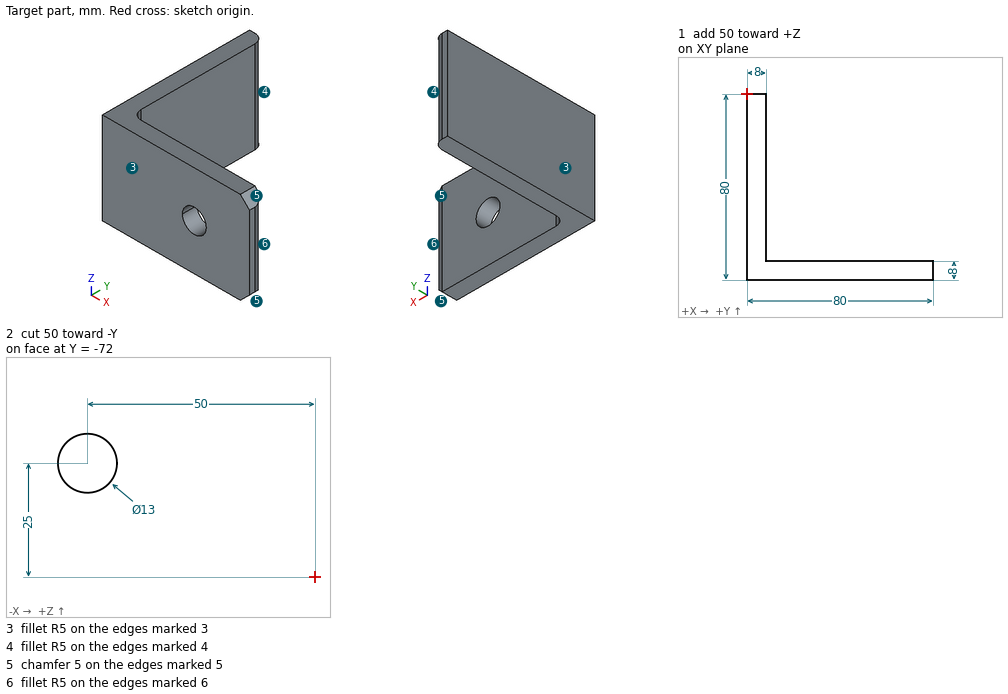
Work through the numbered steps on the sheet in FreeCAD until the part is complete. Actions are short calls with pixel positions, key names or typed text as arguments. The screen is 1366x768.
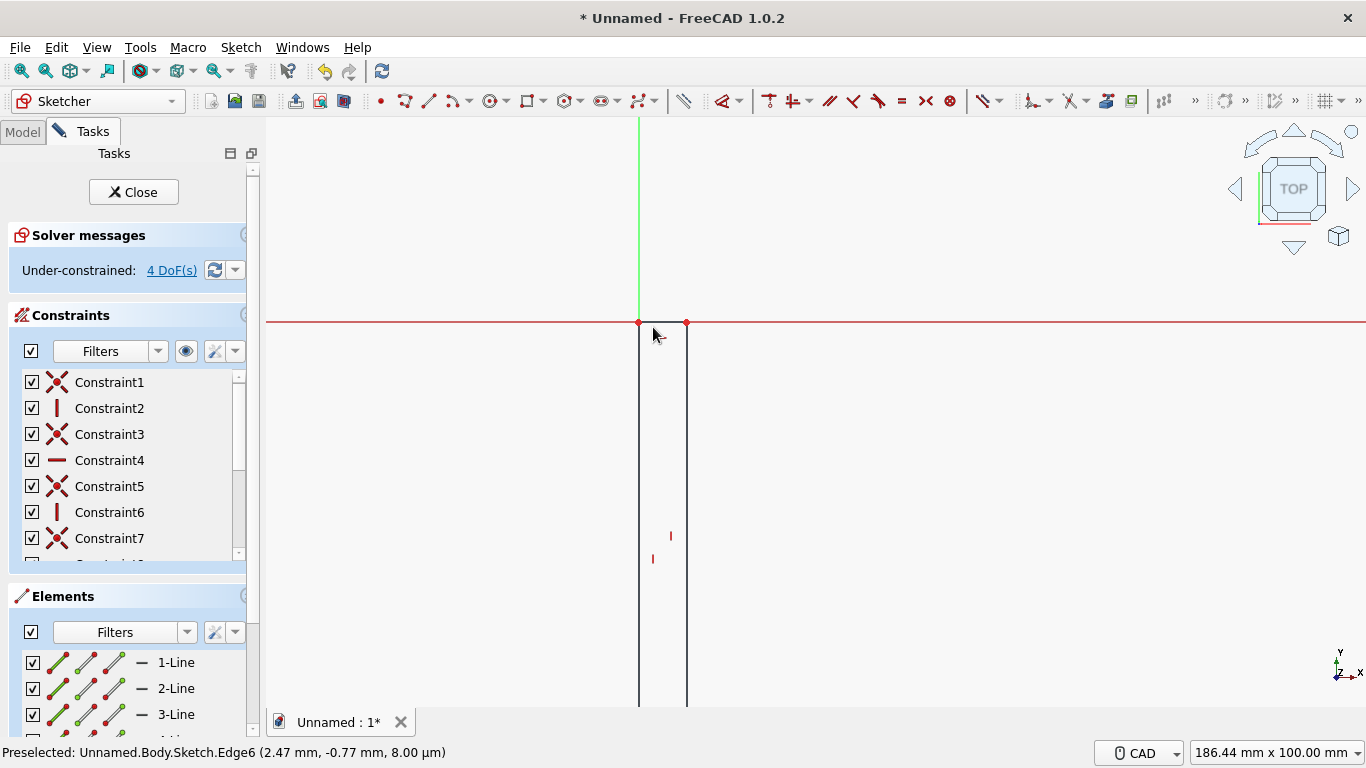
scroll(489, 145, down, 2)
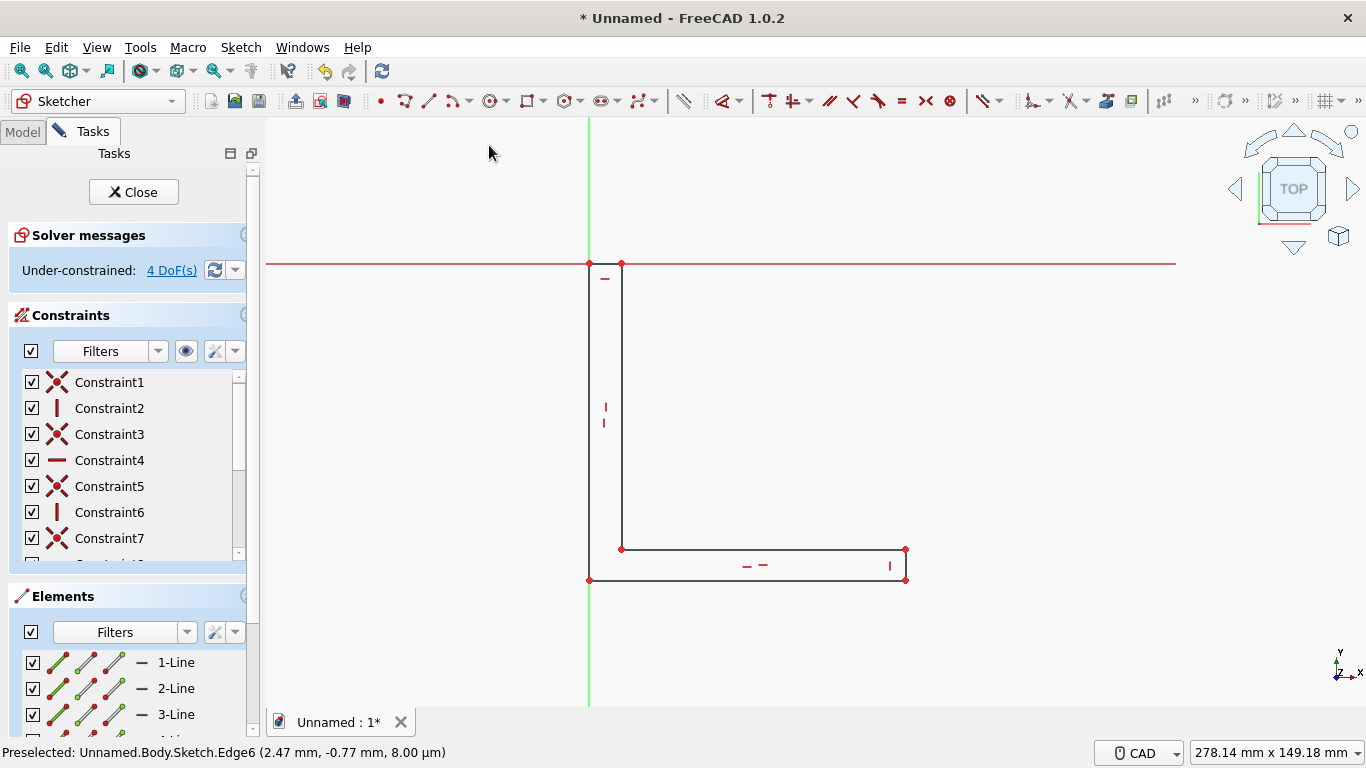
scroll(906, 572, up, 2)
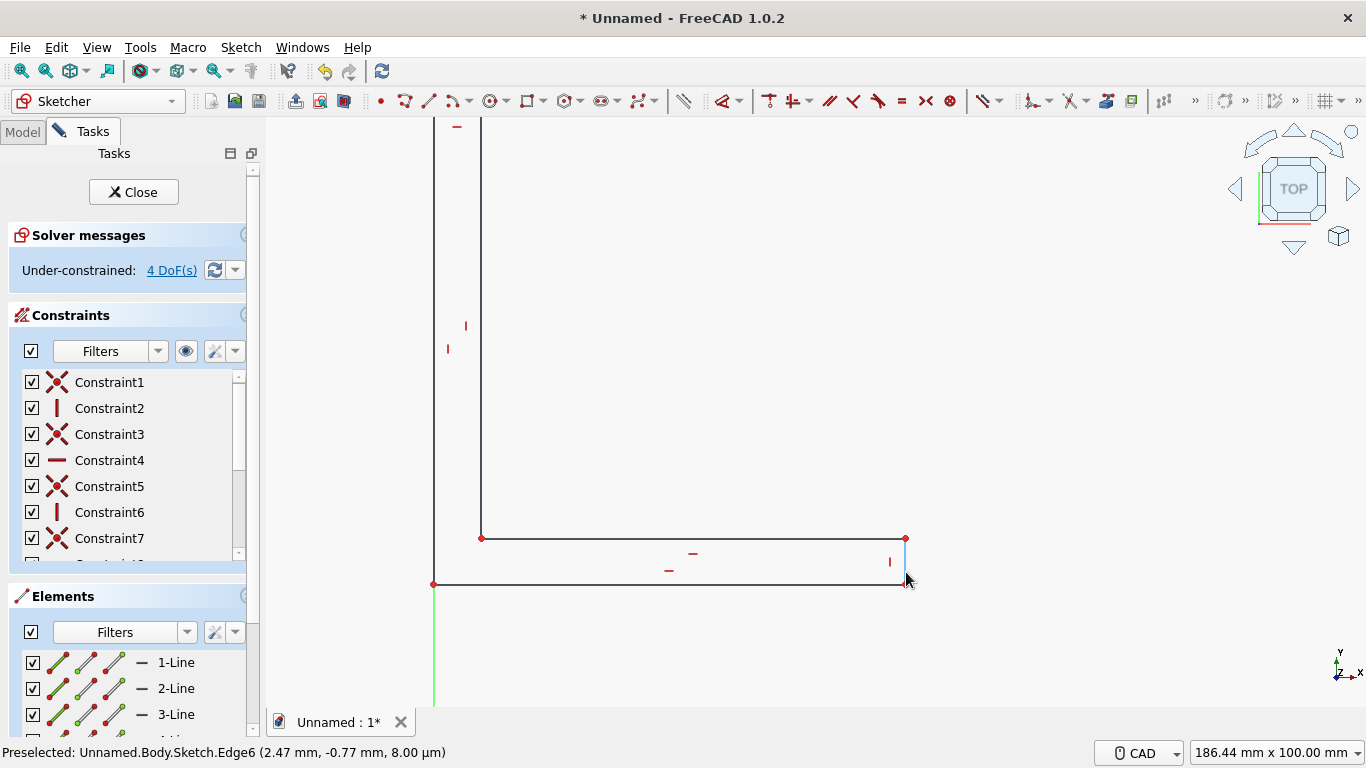
click(905, 571)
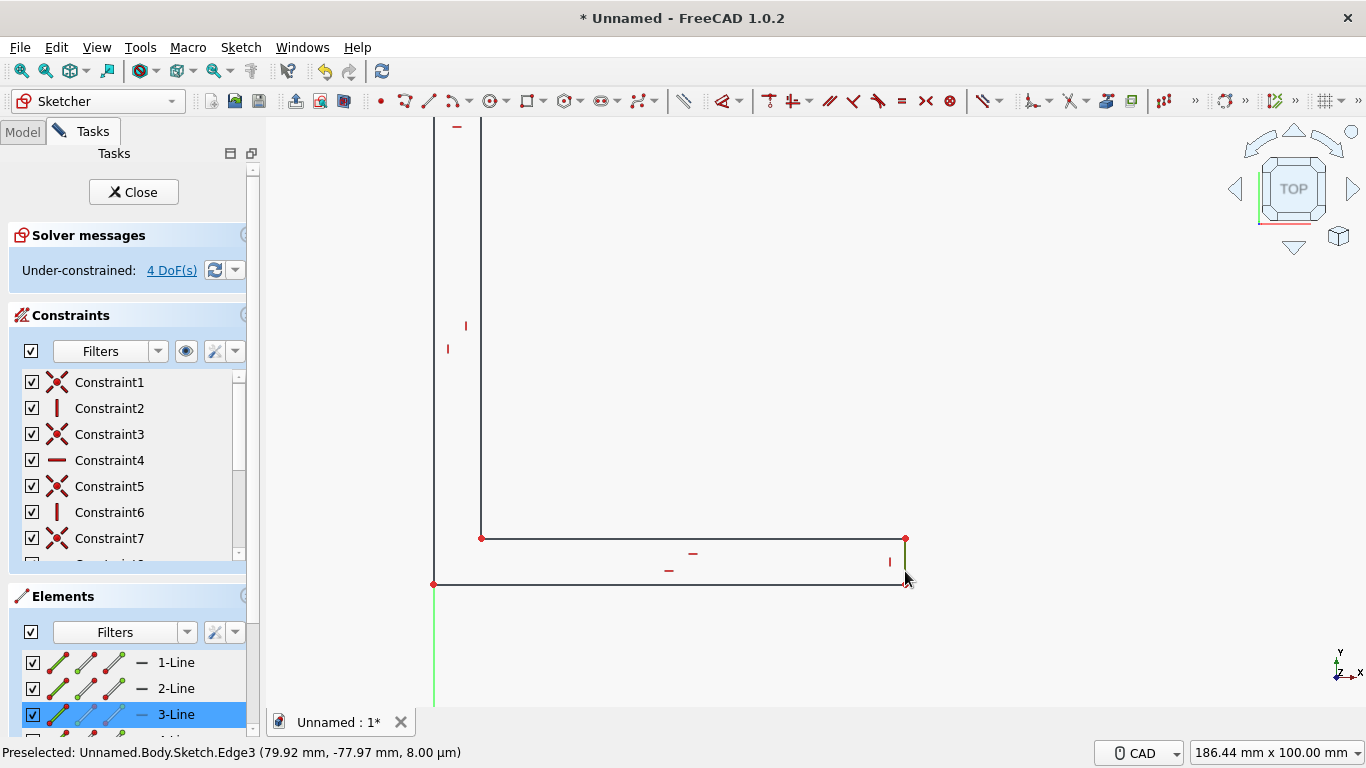
click(742, 102)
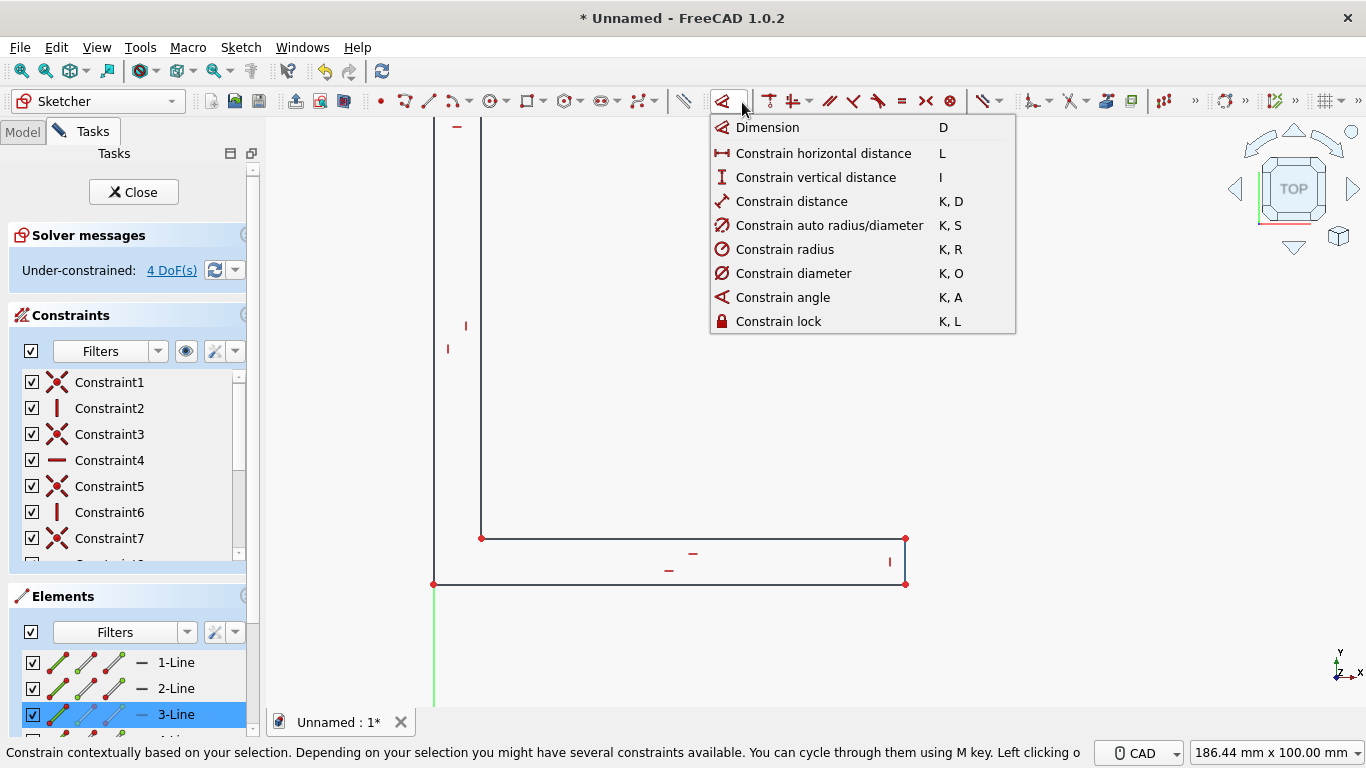
click(863, 177)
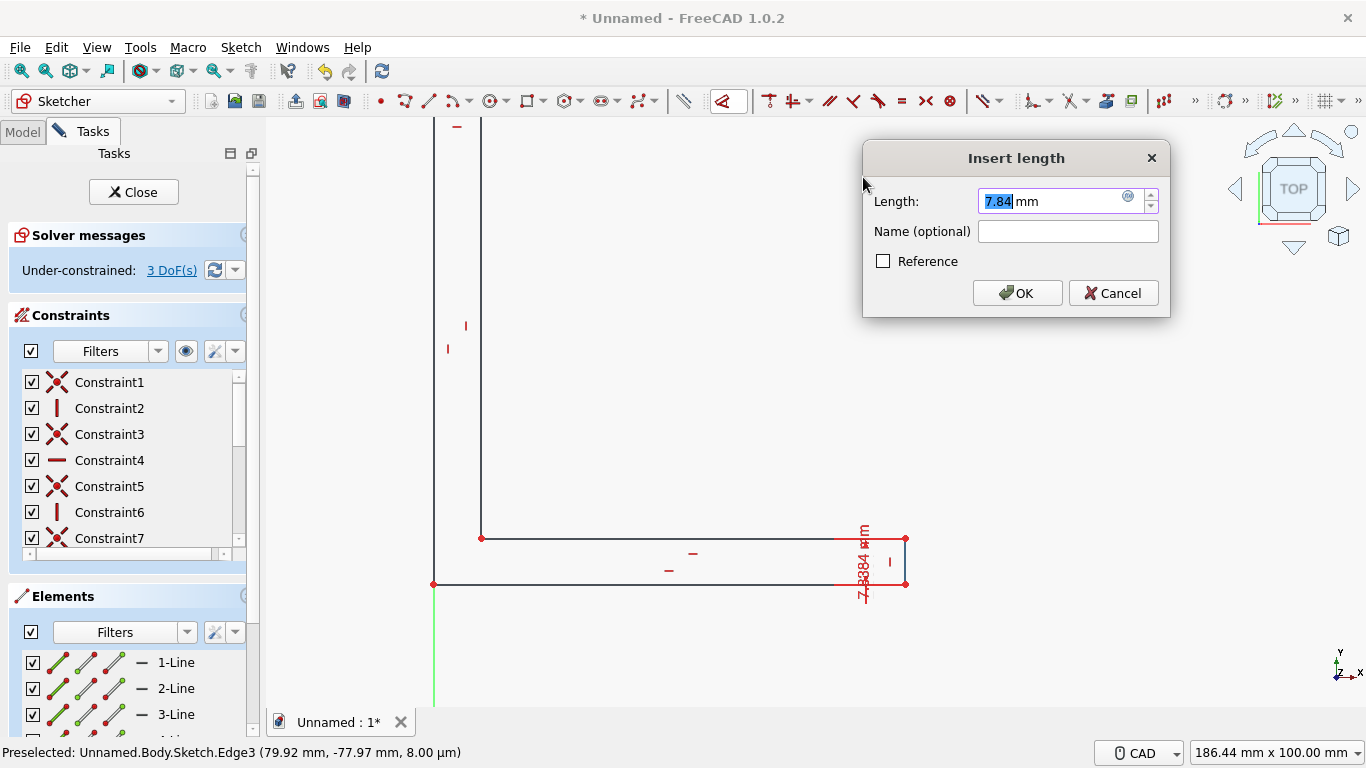
text(8)
key(Return)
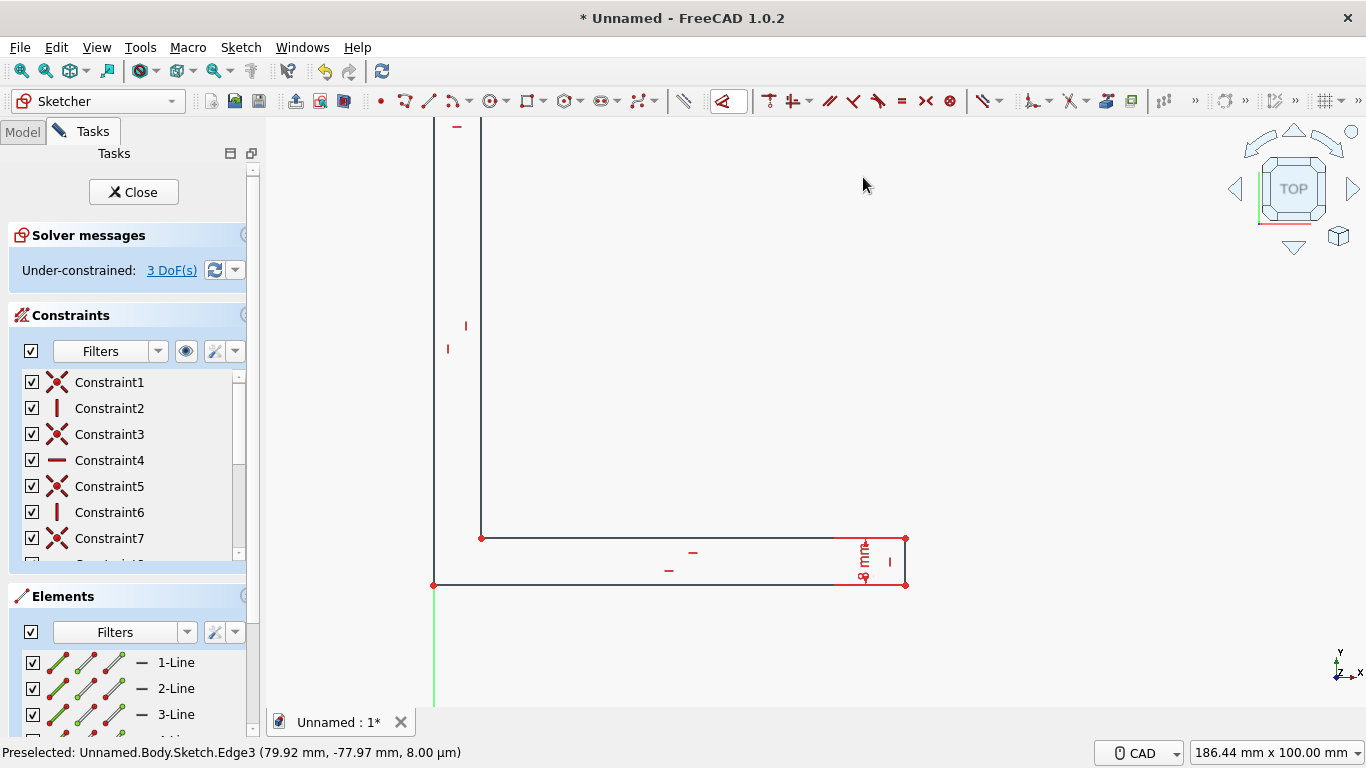
scroll(1100, 679, down, 1)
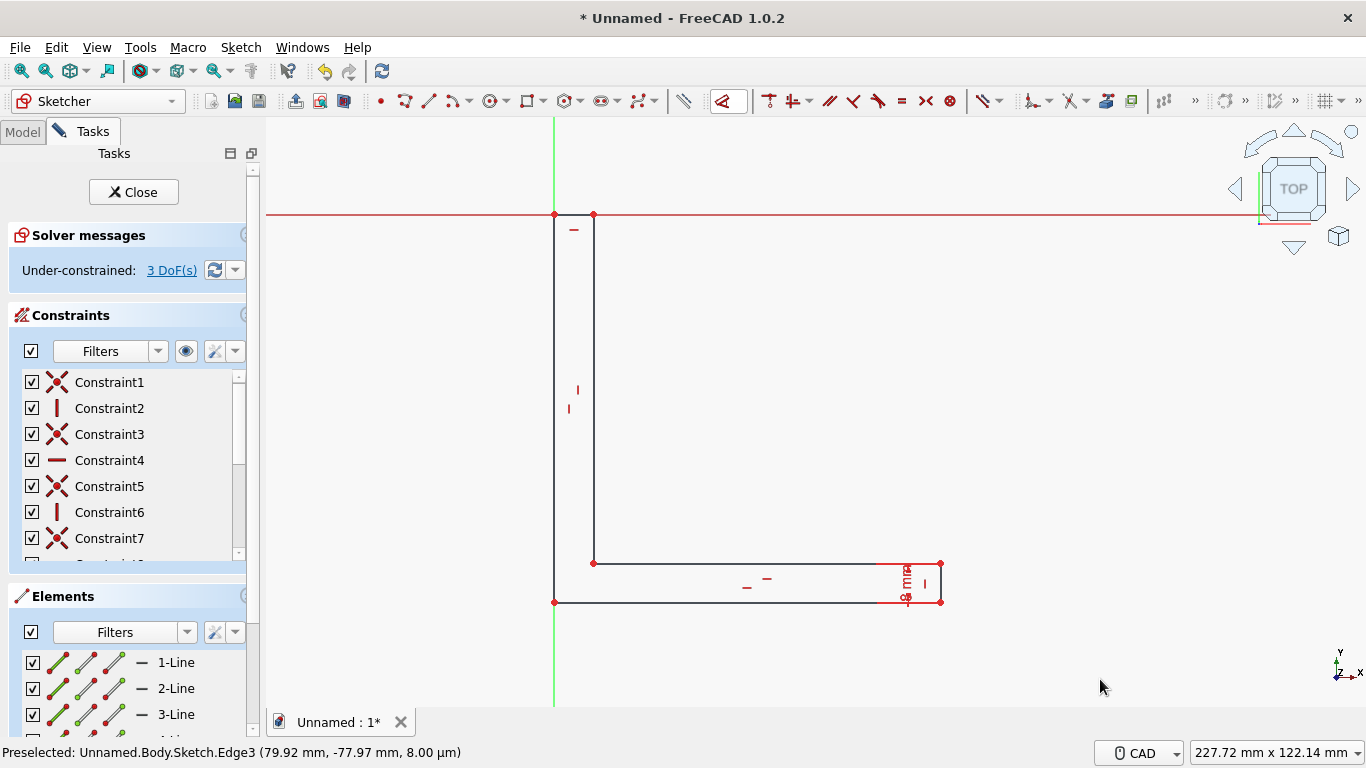
click(582, 215)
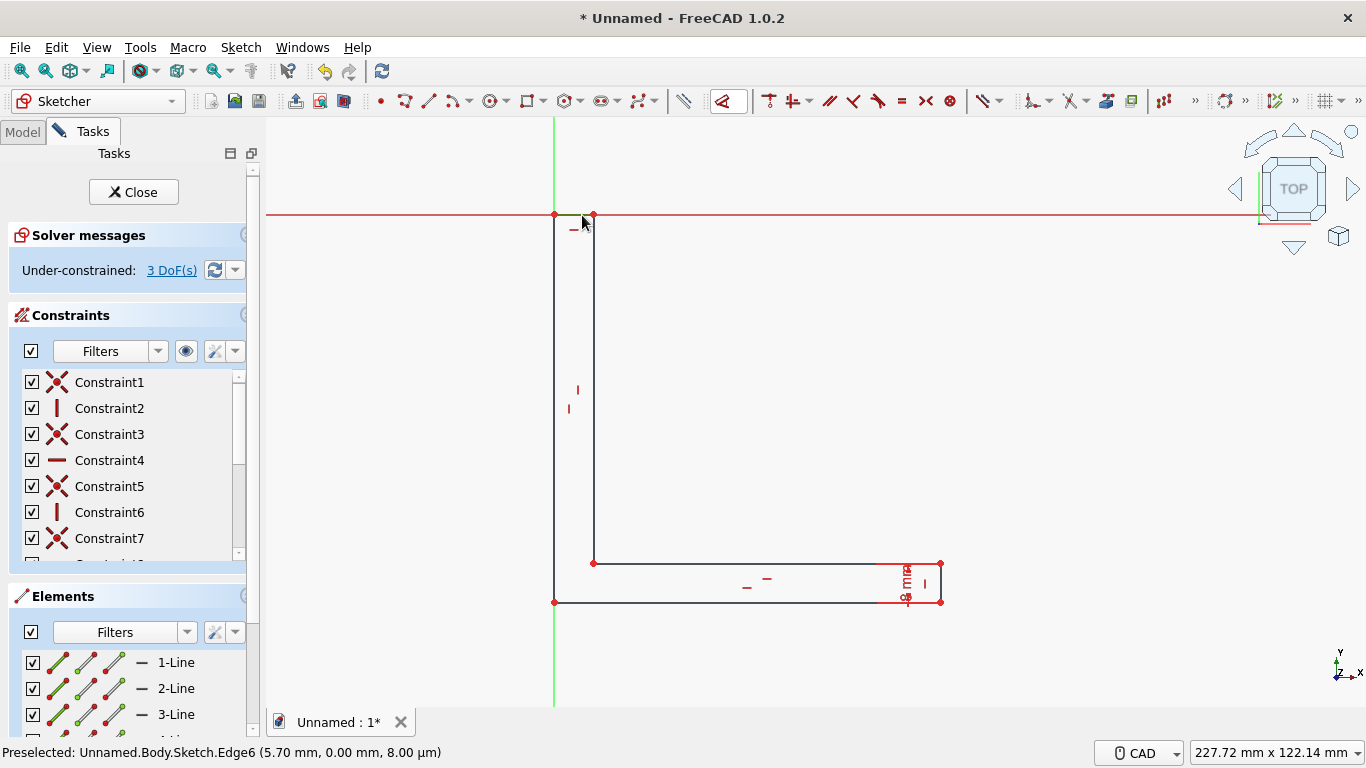
key(l)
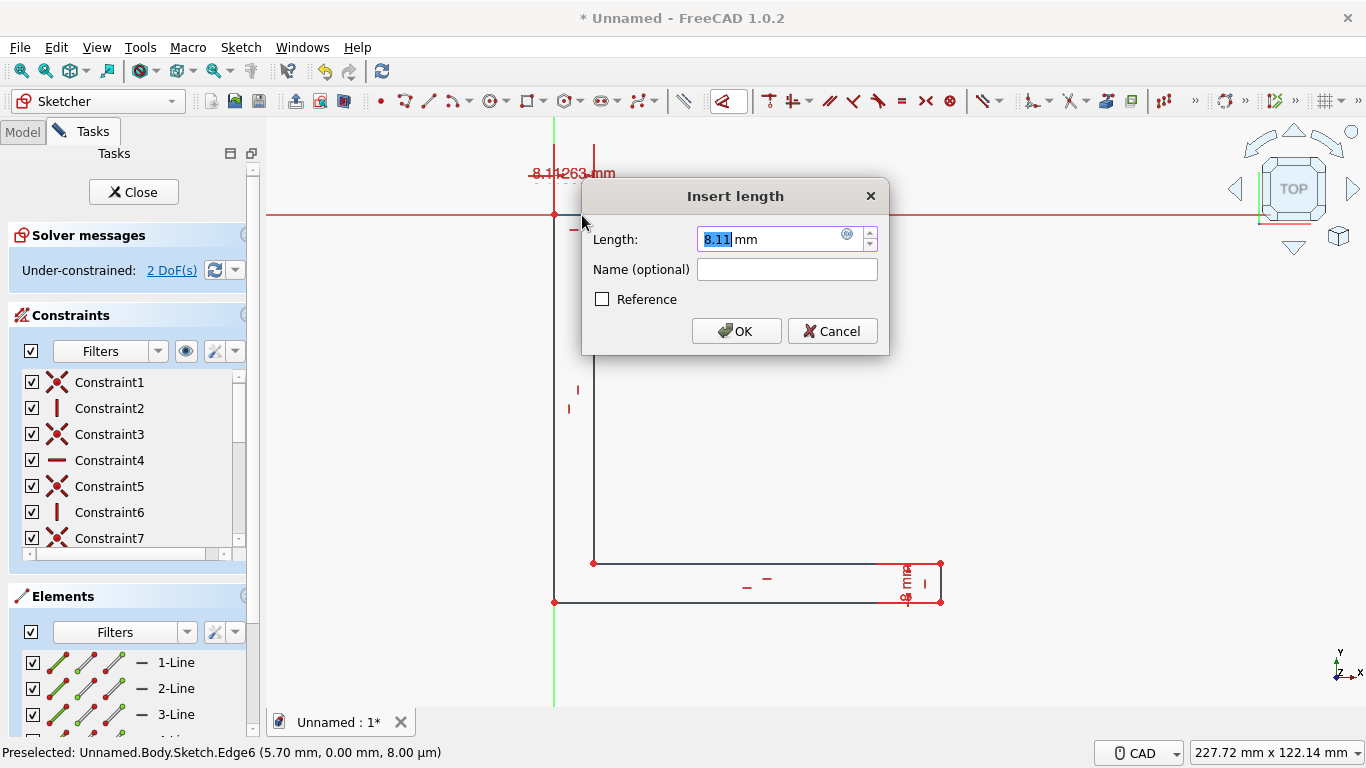
text(8)
key(Return)